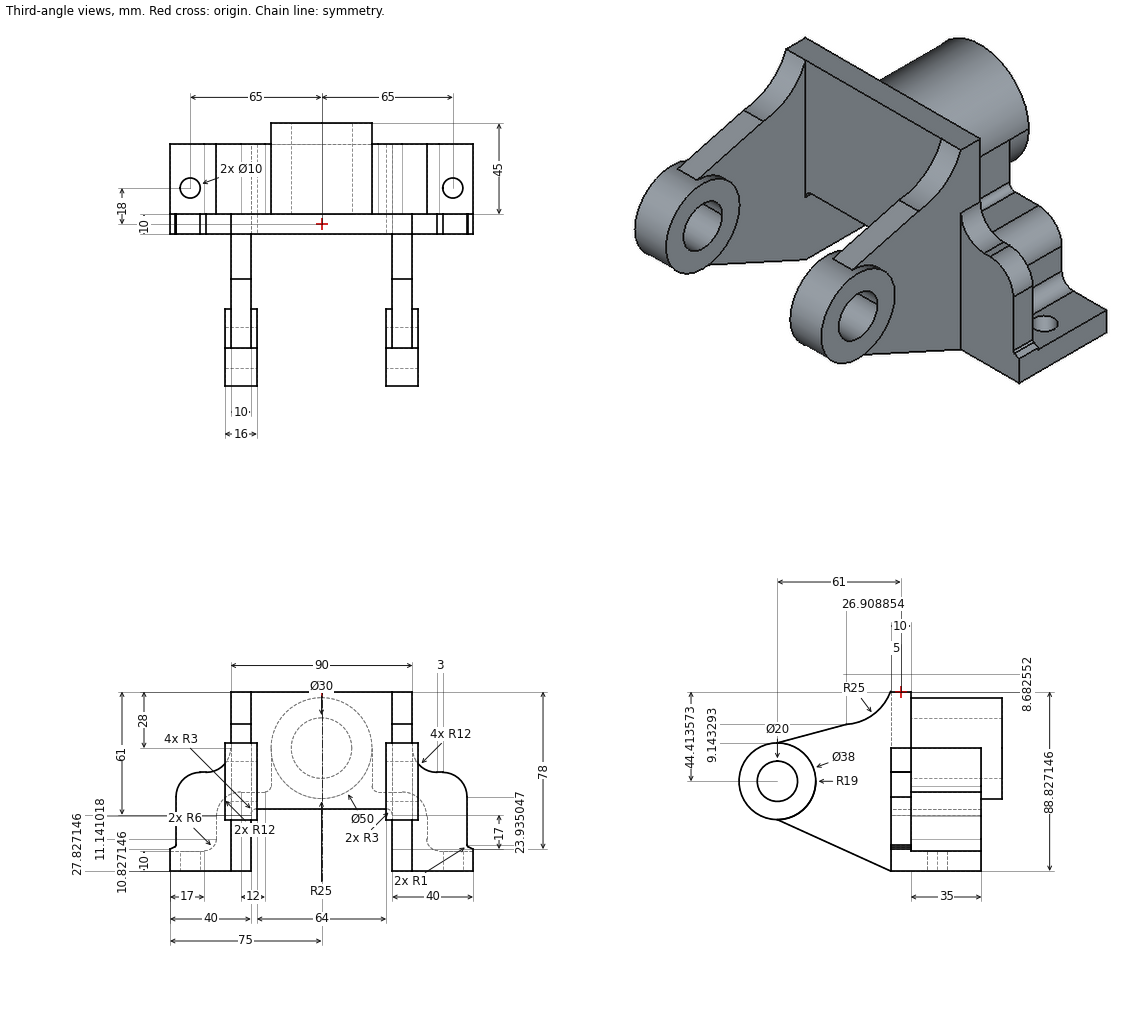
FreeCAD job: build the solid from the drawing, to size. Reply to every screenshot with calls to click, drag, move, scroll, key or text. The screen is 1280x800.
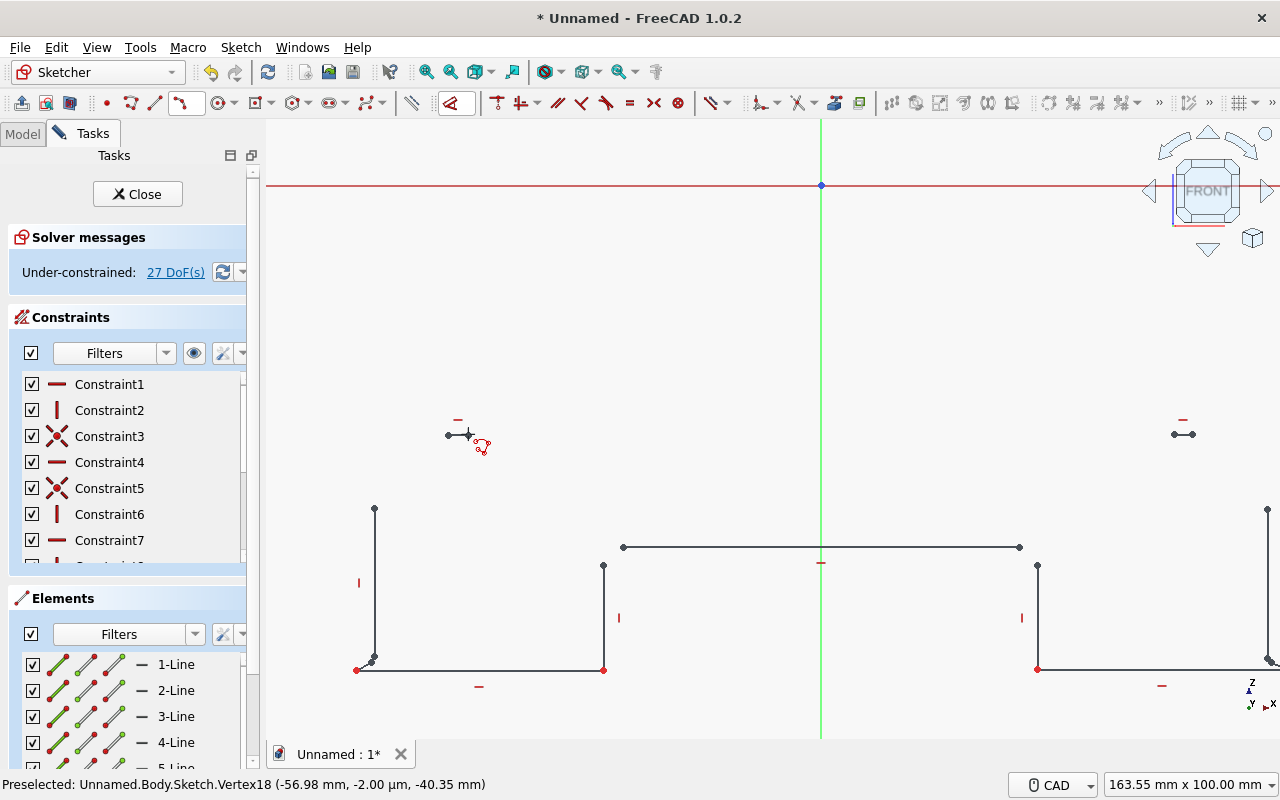
click(542, 359)
click(542, 186)
click(1100, 195)
click(1100, 359)
right_click(1100, 359)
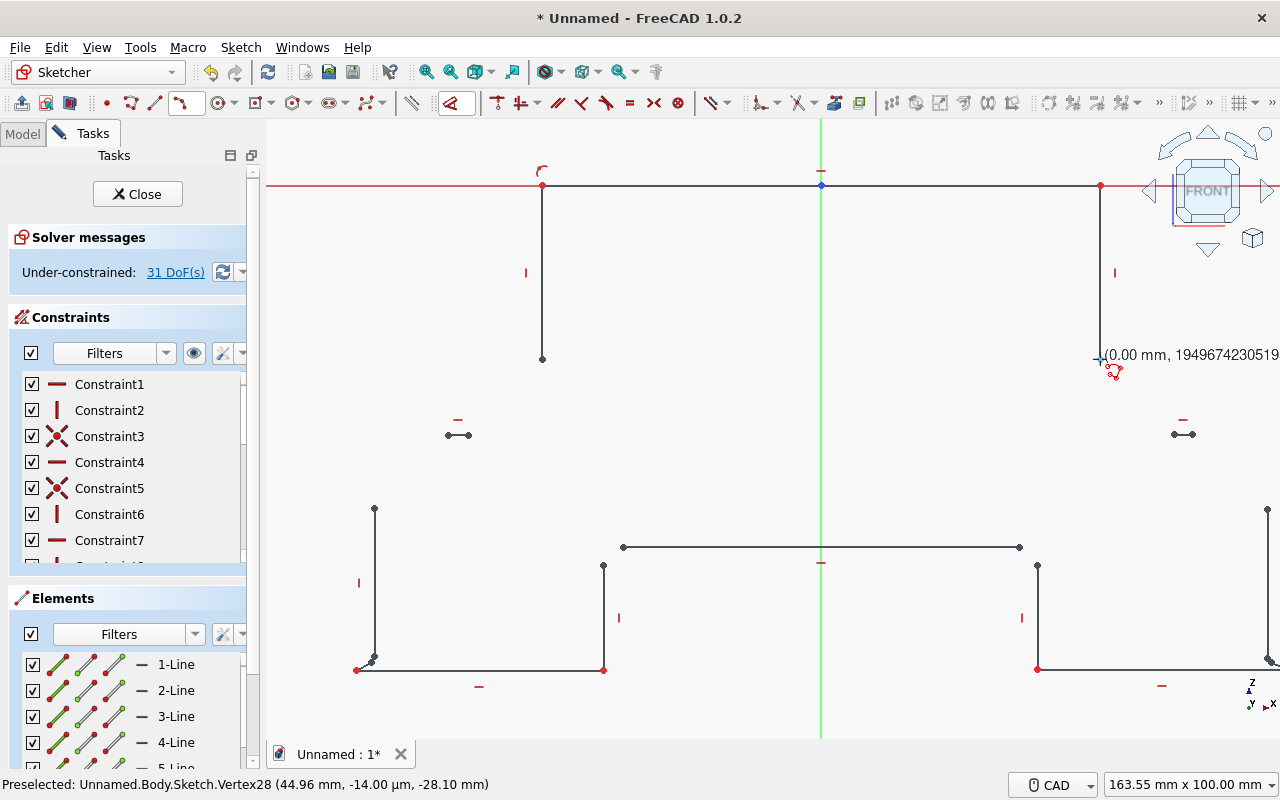
key(g)
key(3)
key(a)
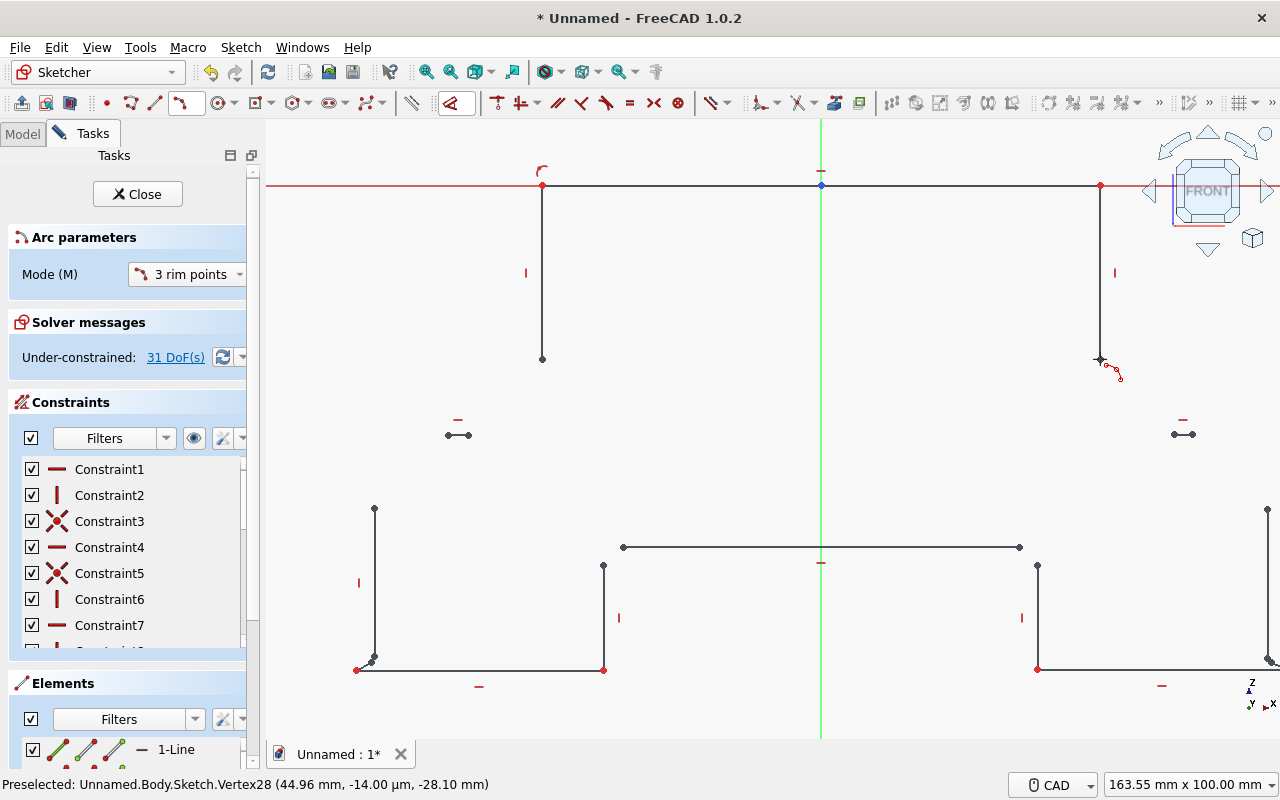
scroll(467, 432, down, 2)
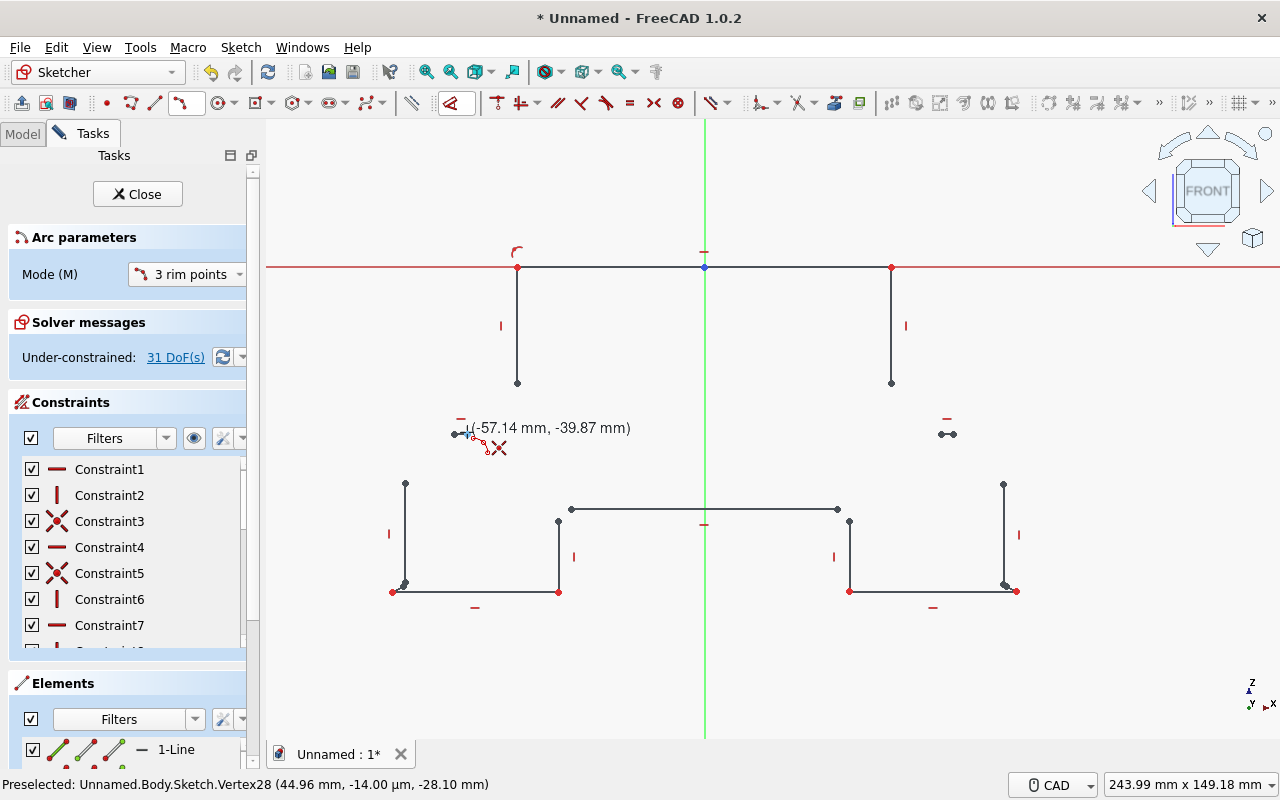
scroll(954, 433, up, 5)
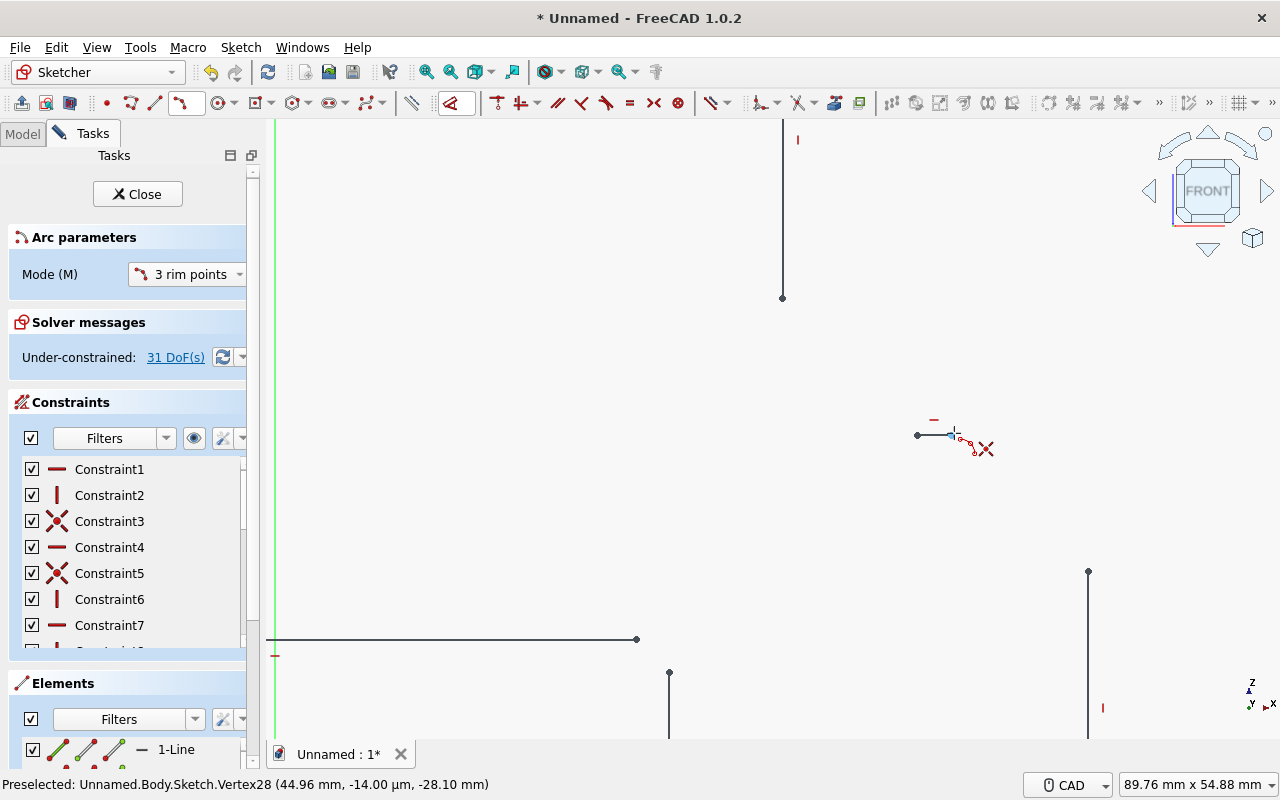
click(952, 435)
click(1088, 571)
click(1048, 473)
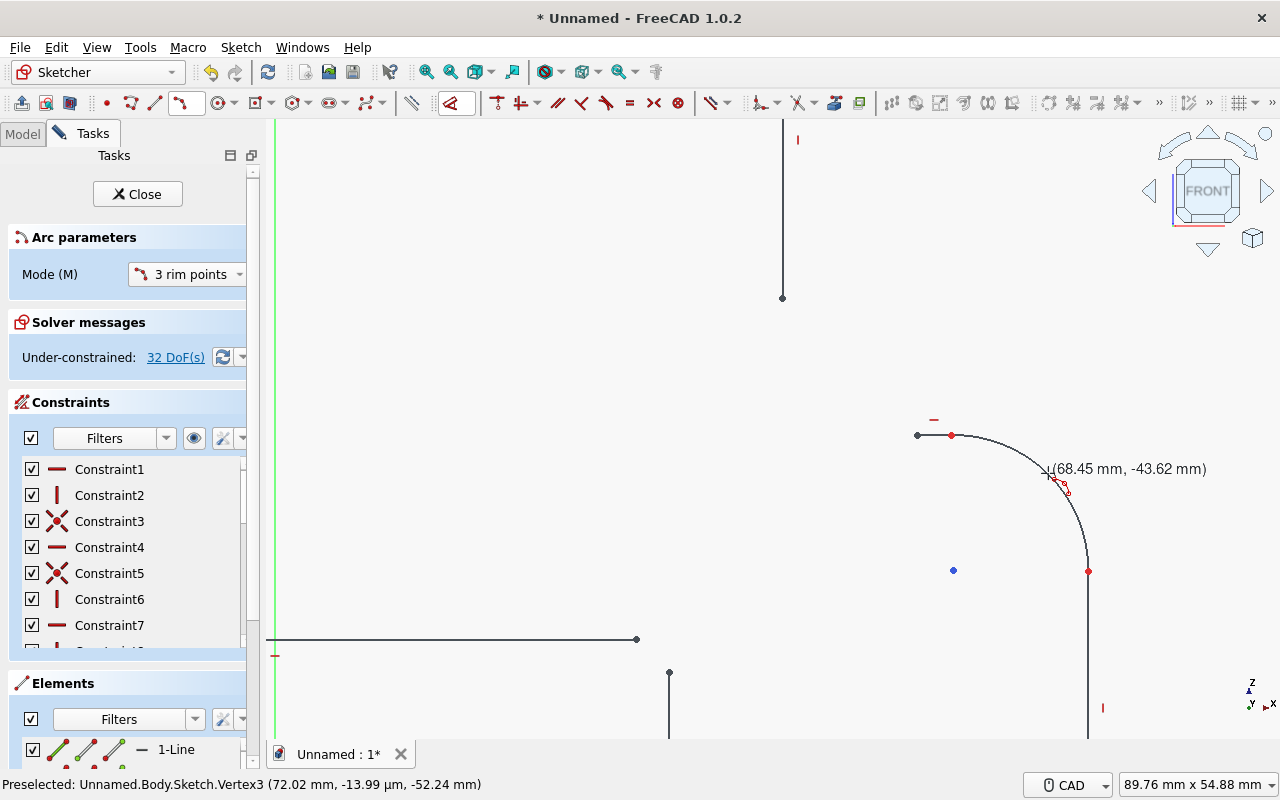
scroll(955, 433, down, 5)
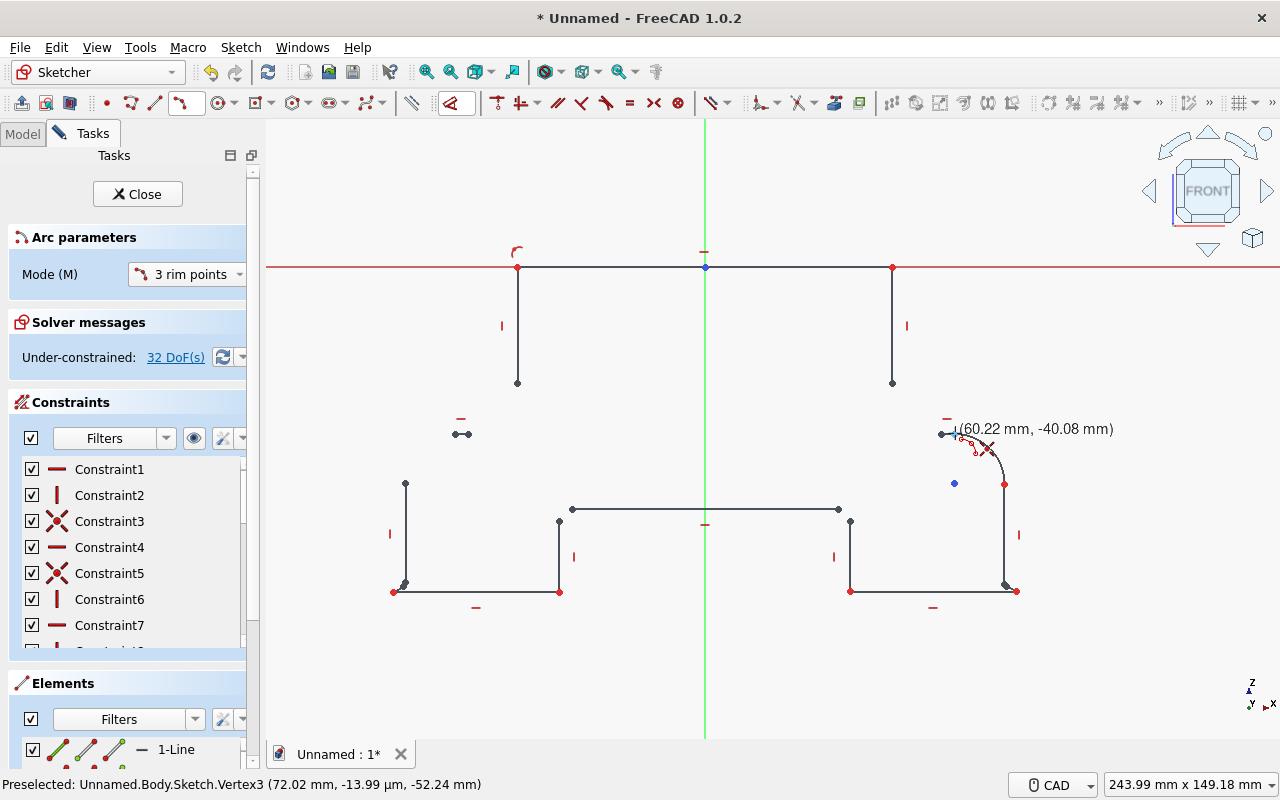
scroll(1004, 583, up, 7)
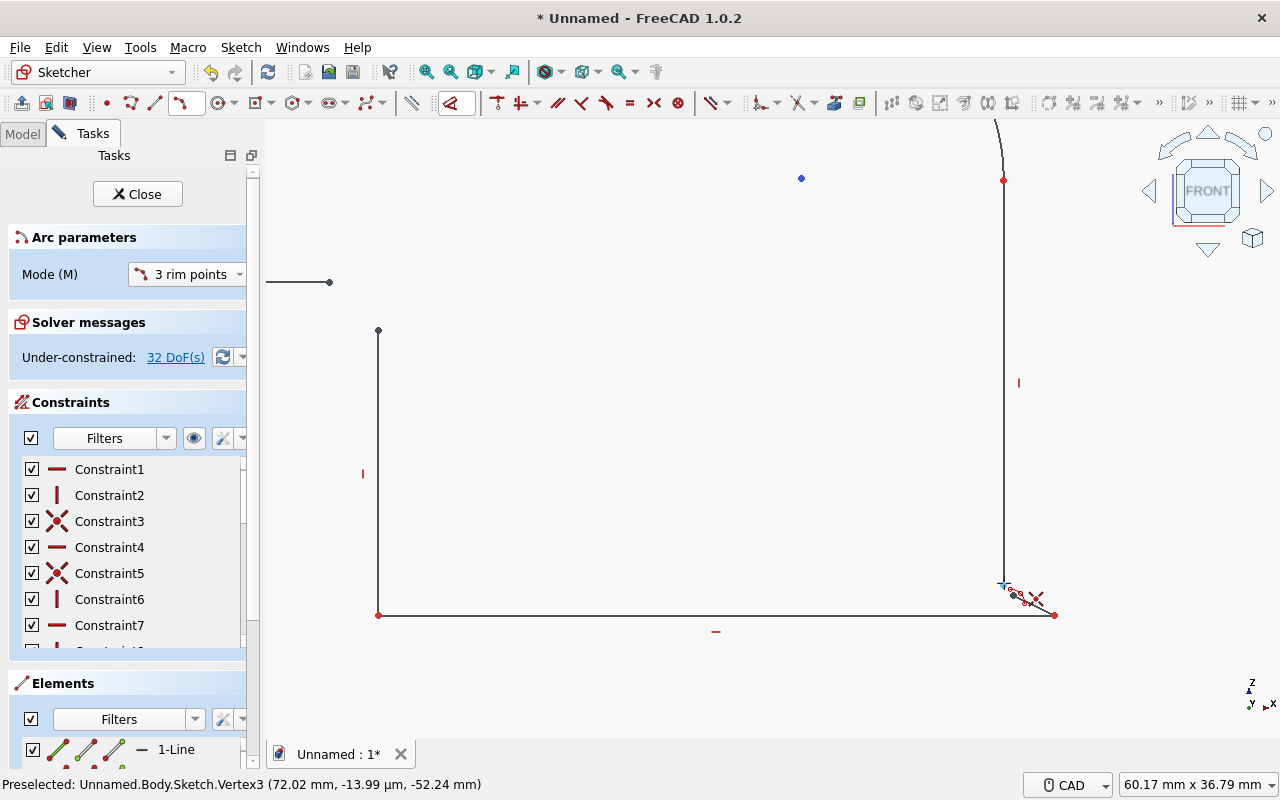
click(1004, 585)
click(1013, 596)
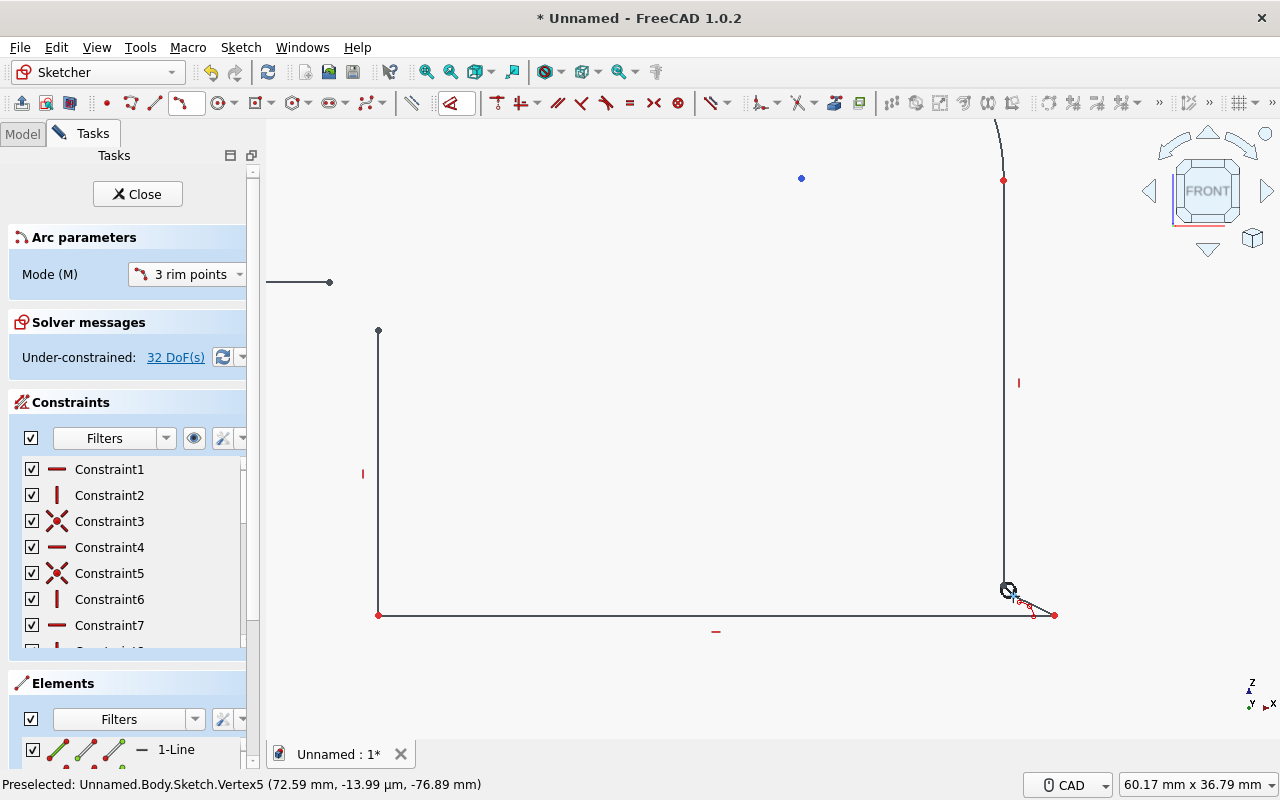
scroll(1006, 589, up, 10)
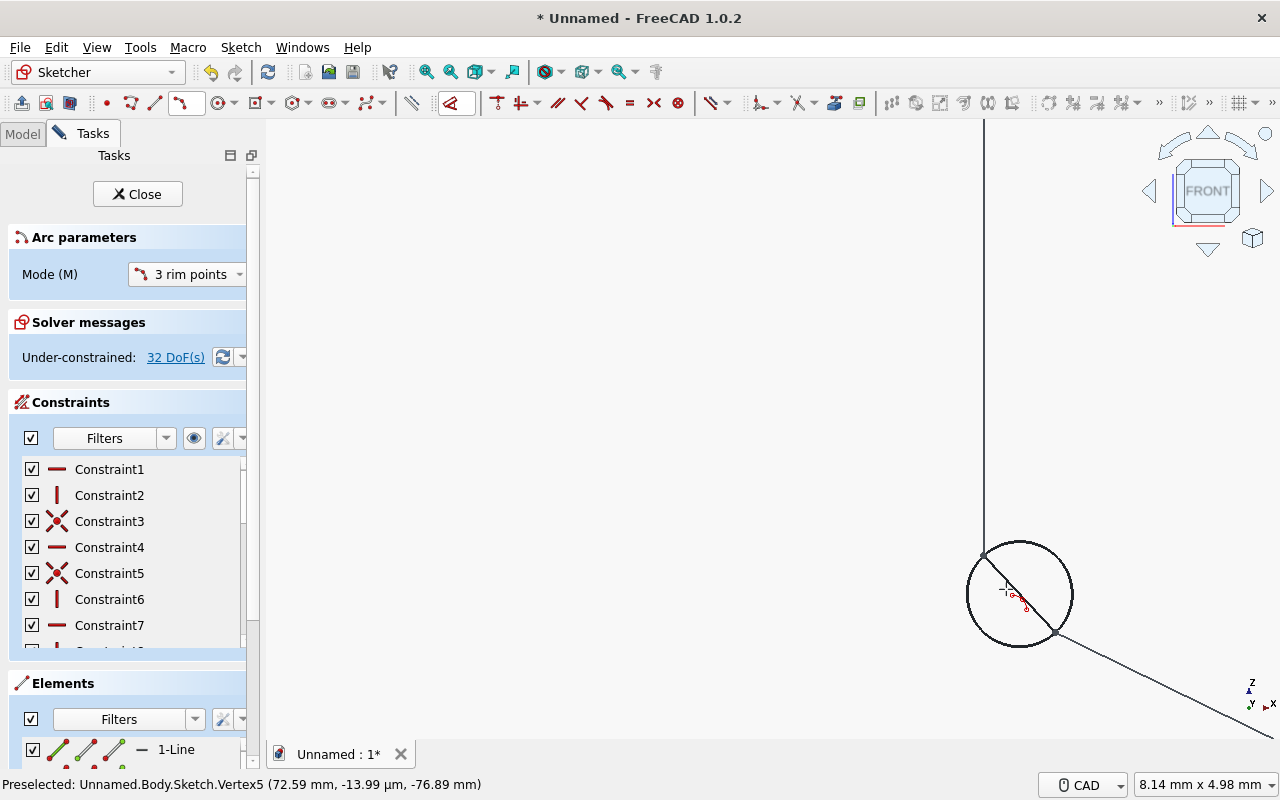
click(1001, 581)